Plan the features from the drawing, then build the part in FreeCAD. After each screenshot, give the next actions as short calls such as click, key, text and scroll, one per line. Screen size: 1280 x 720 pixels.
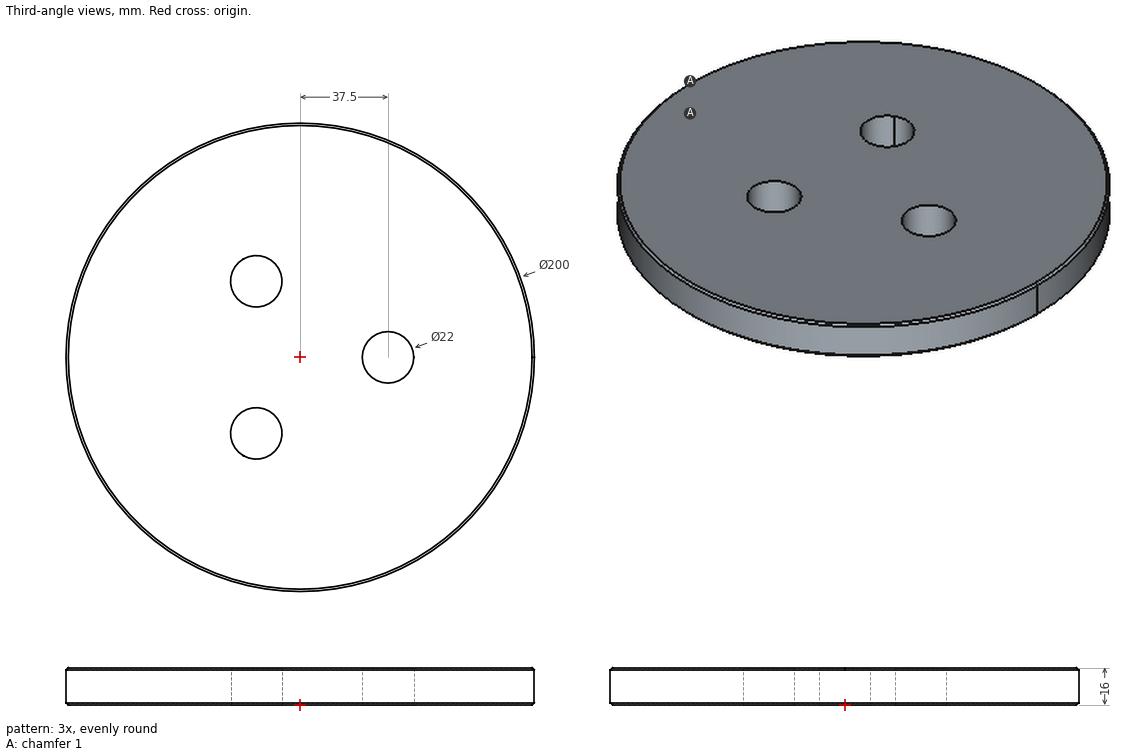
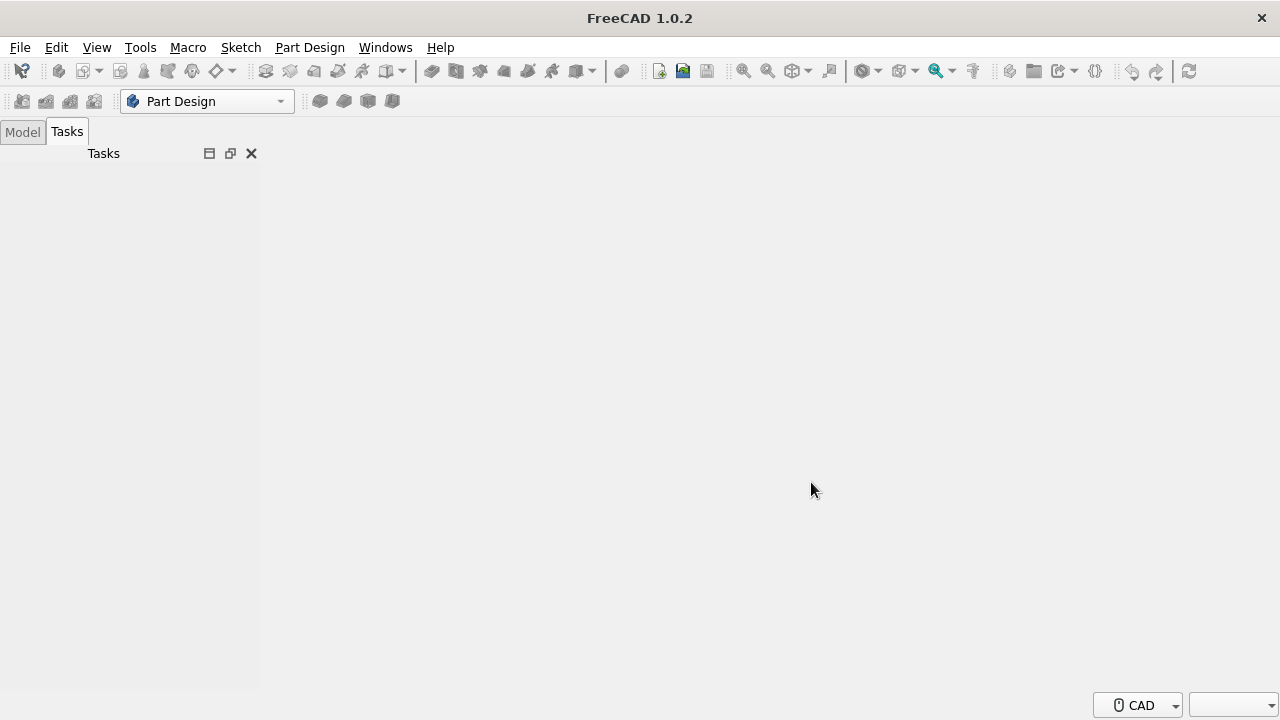
click(660, 72)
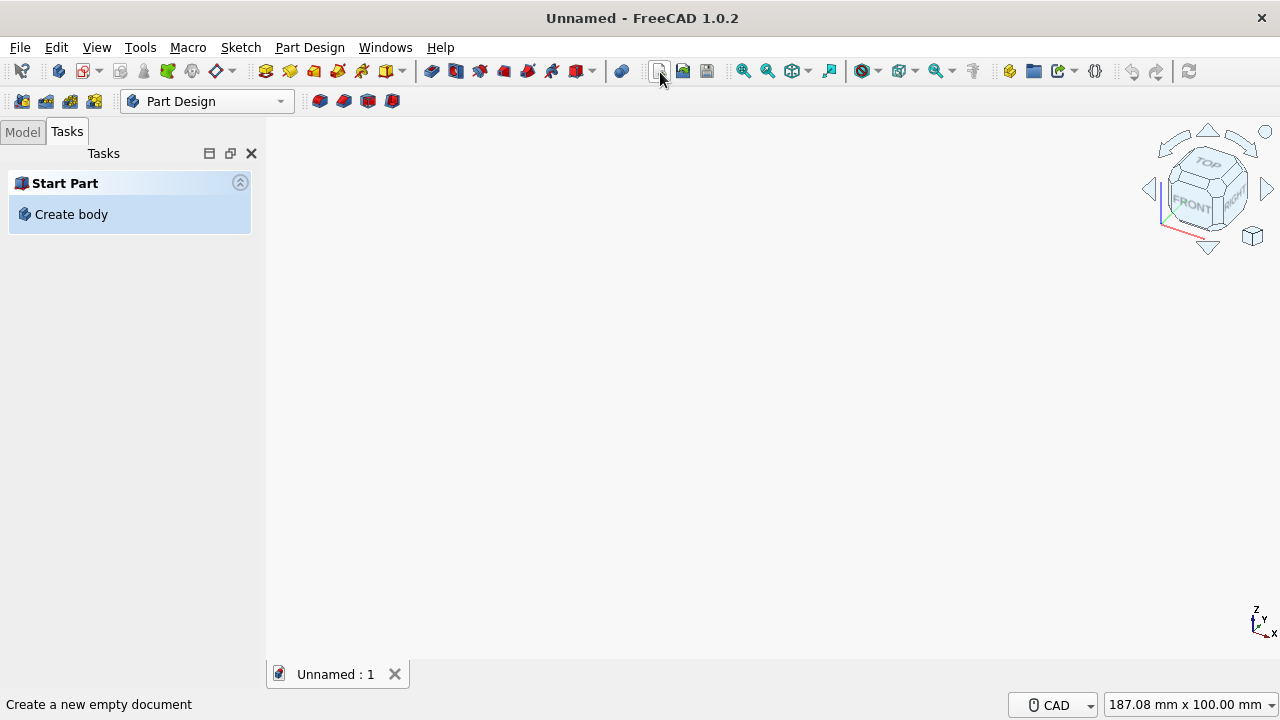
click(84, 72)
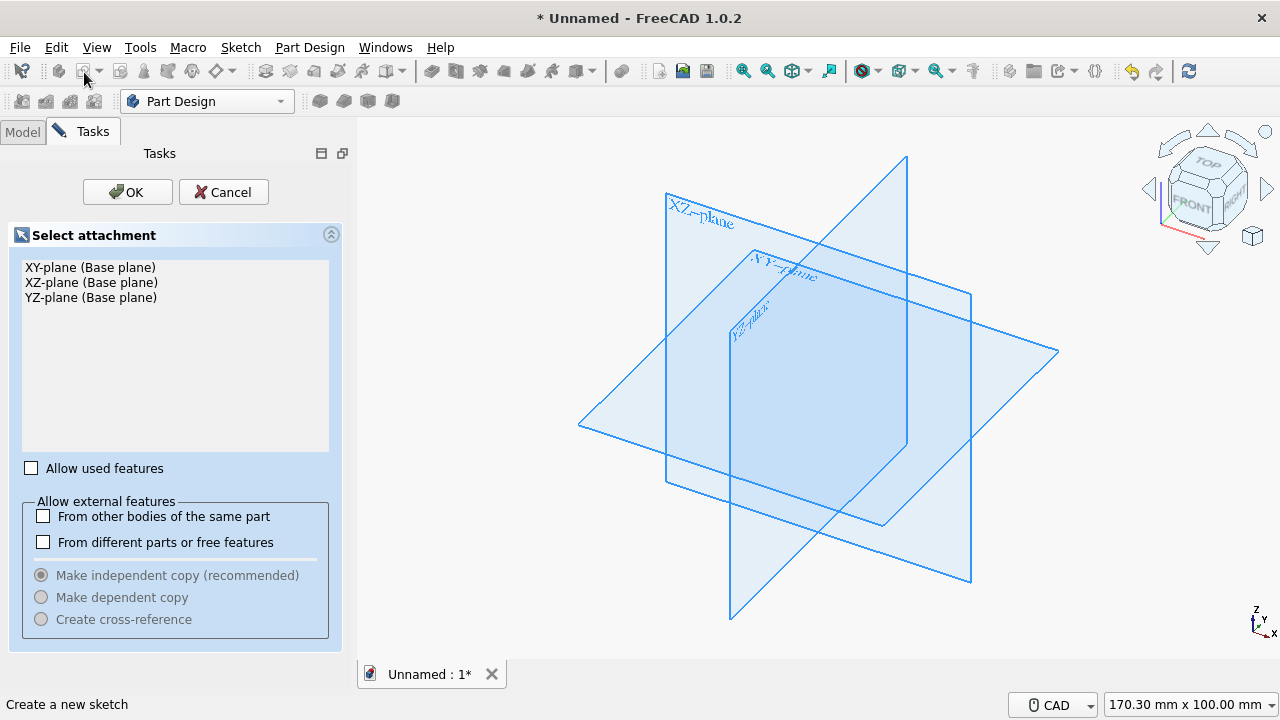
click(82, 268)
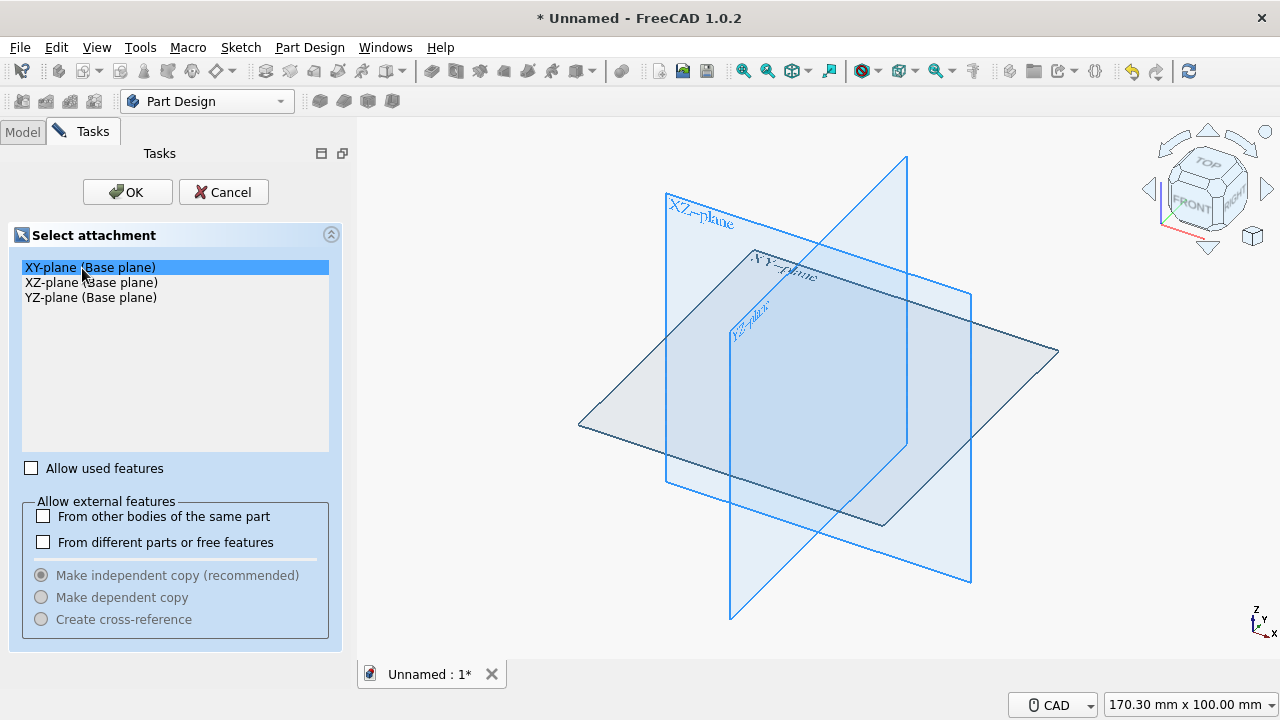
click(128, 192)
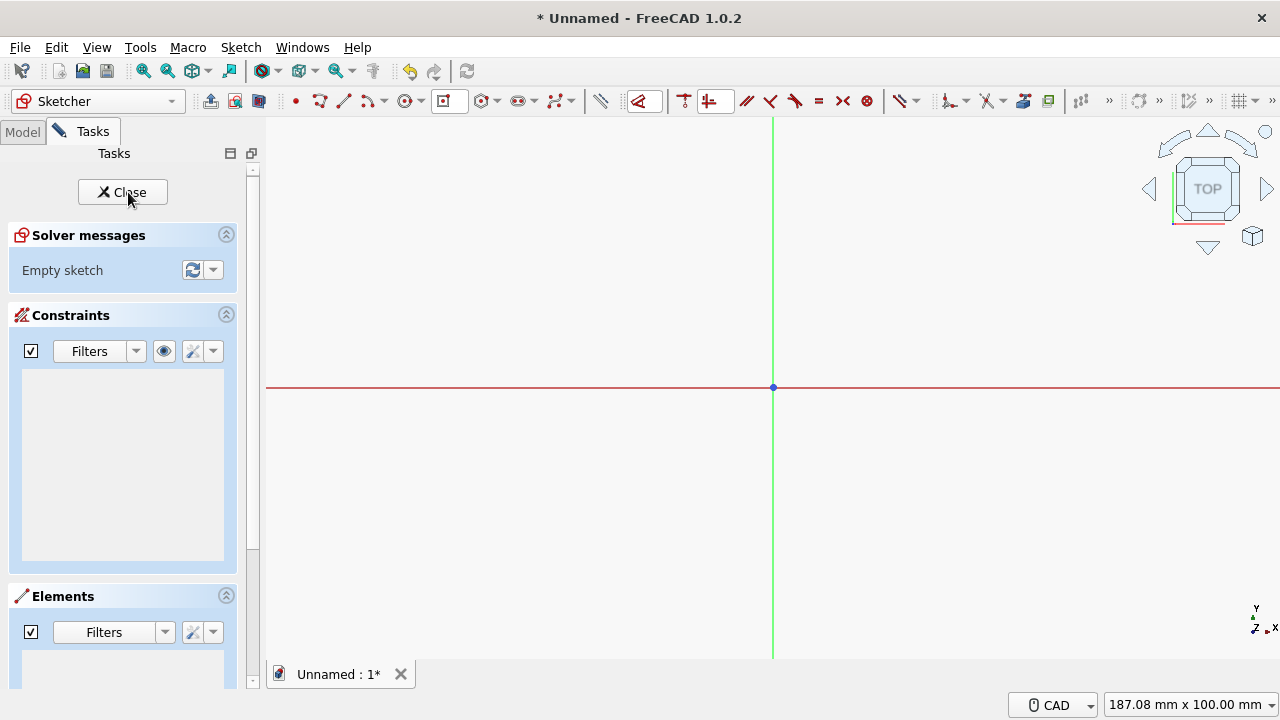
scroll(675, 388, down, 6)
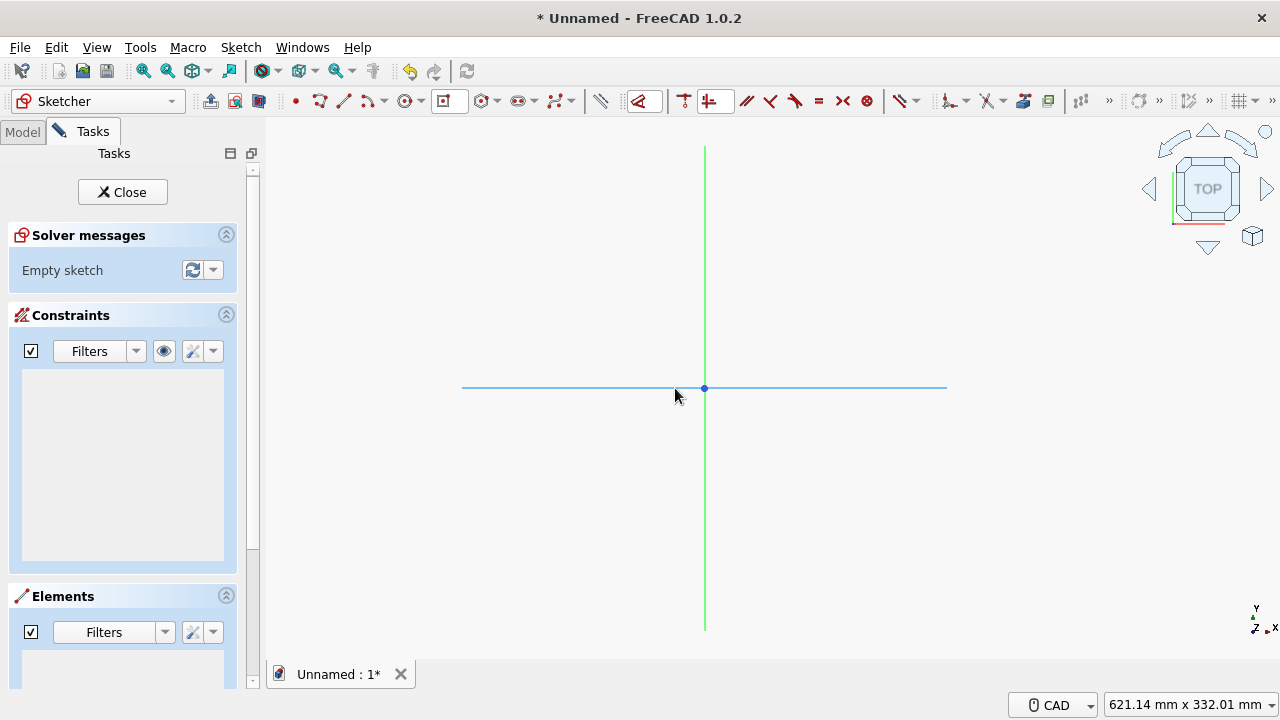
click(406, 102)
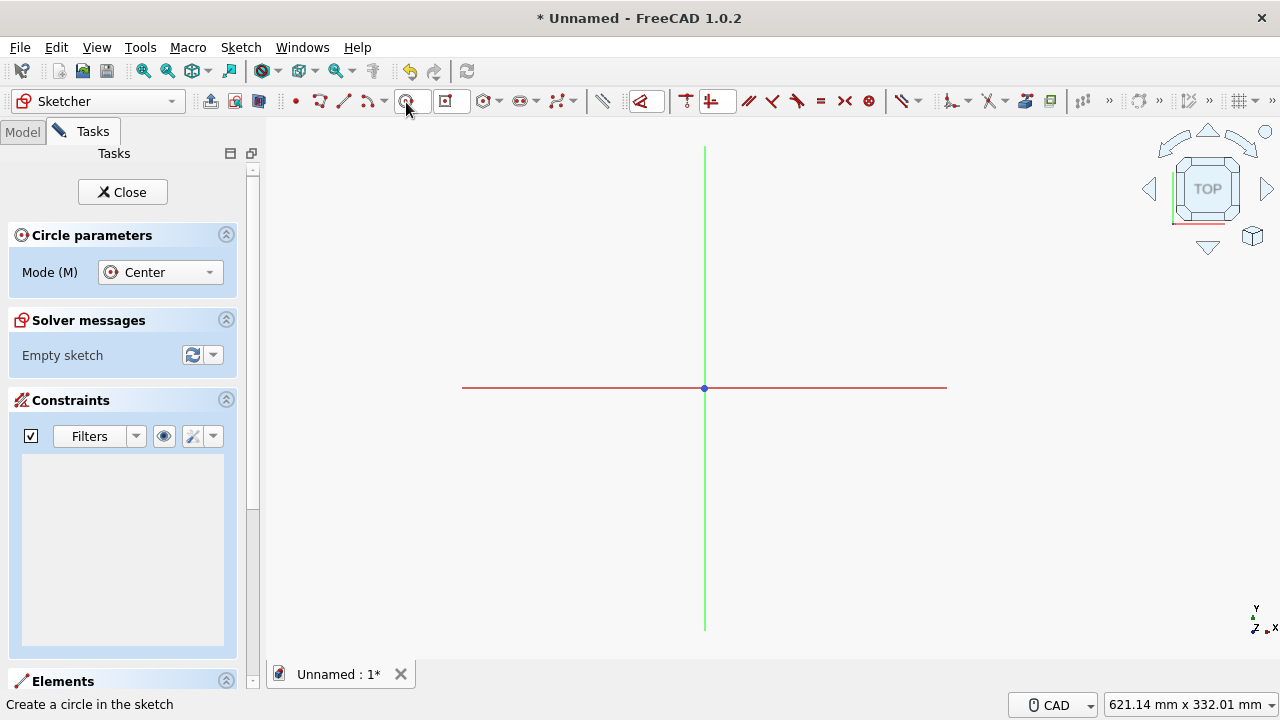
click(705, 388)
click(820, 273)
key(Escape)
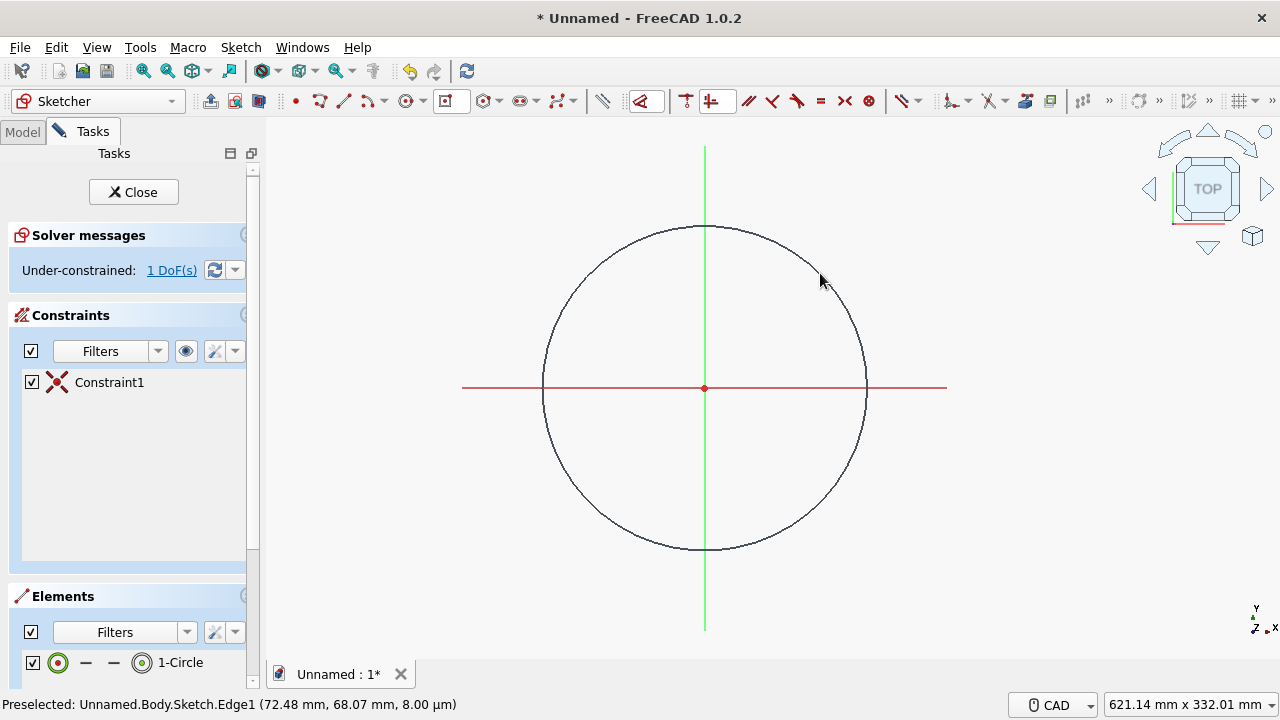
key(d)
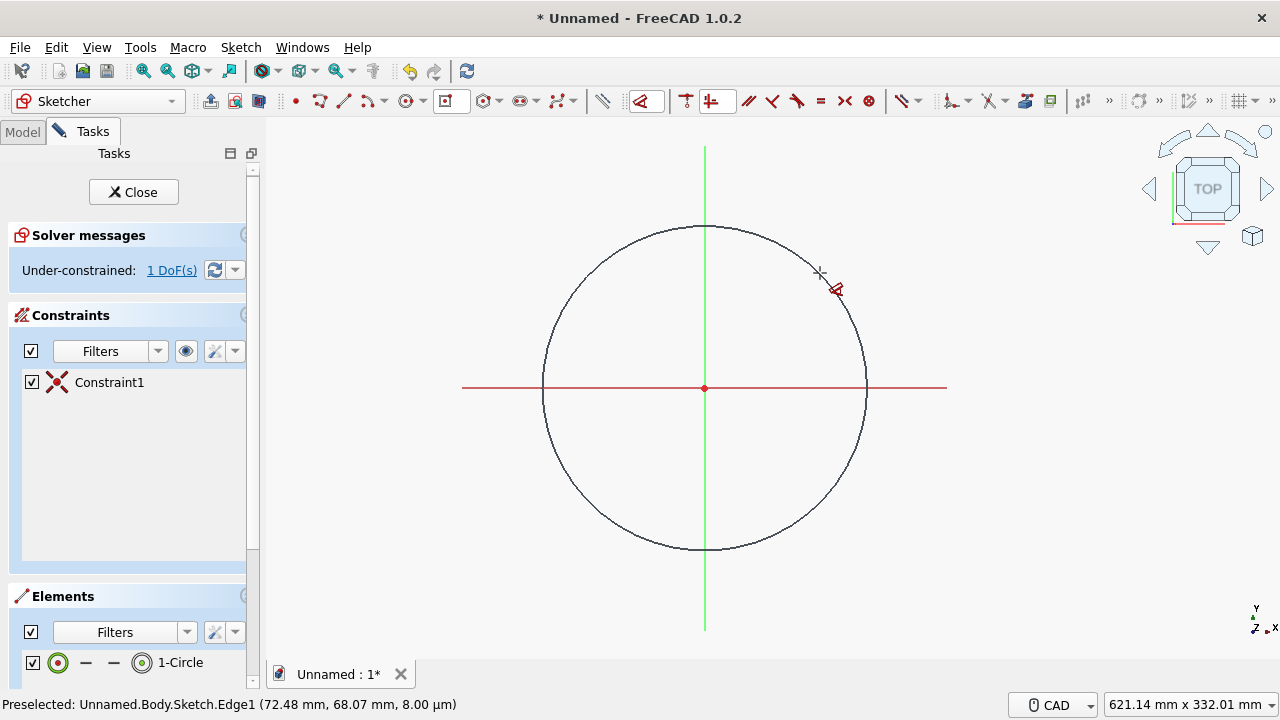
click(819, 273)
click(842, 250)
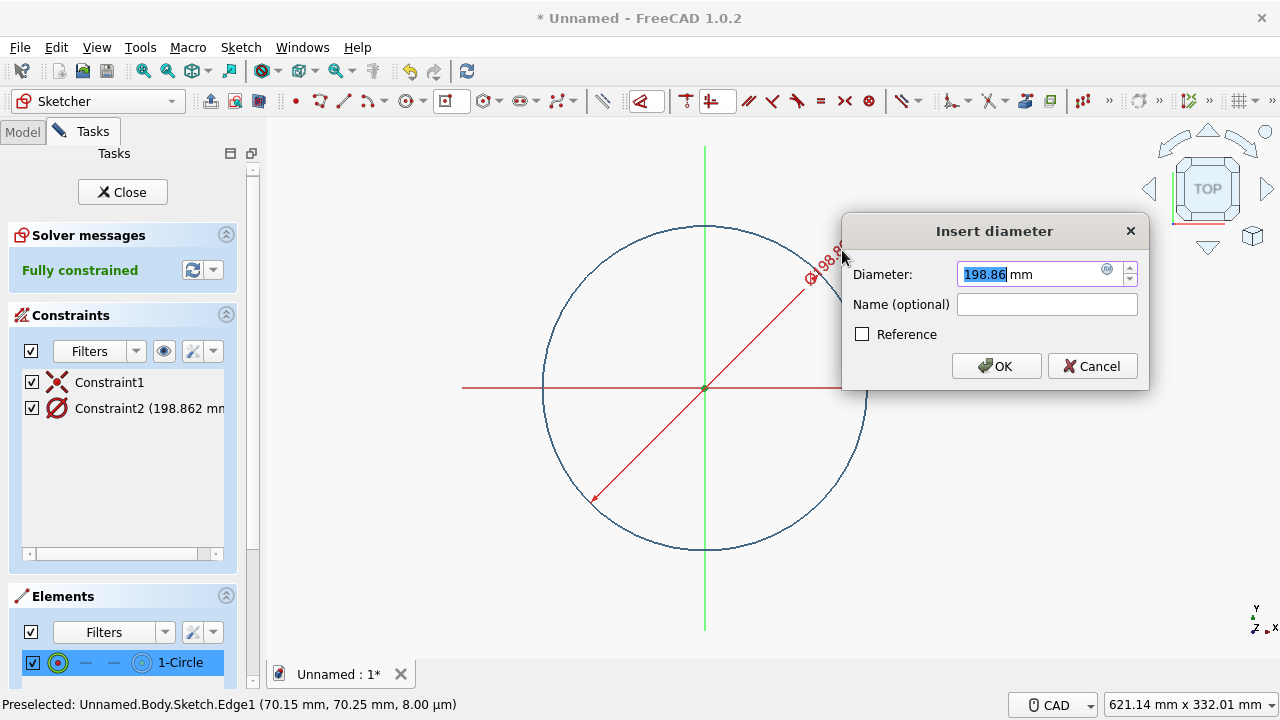
text(200)
key(Return)
key(Escape)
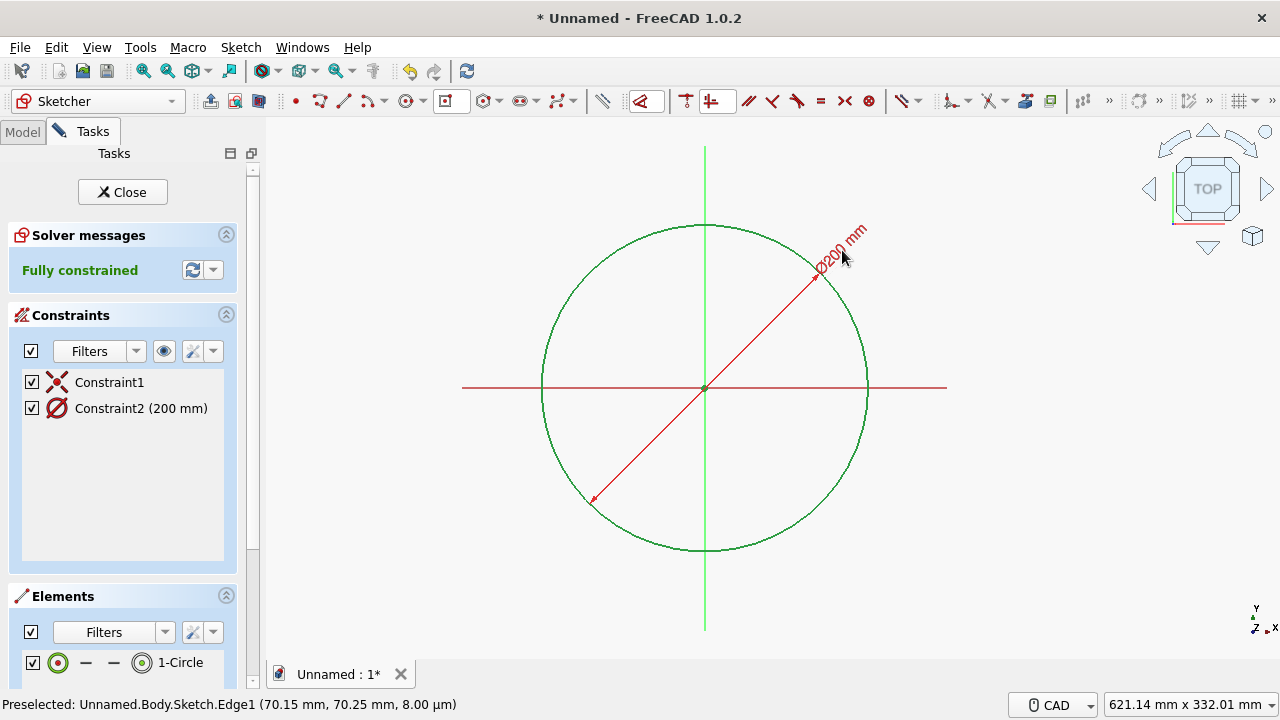
click(123, 192)